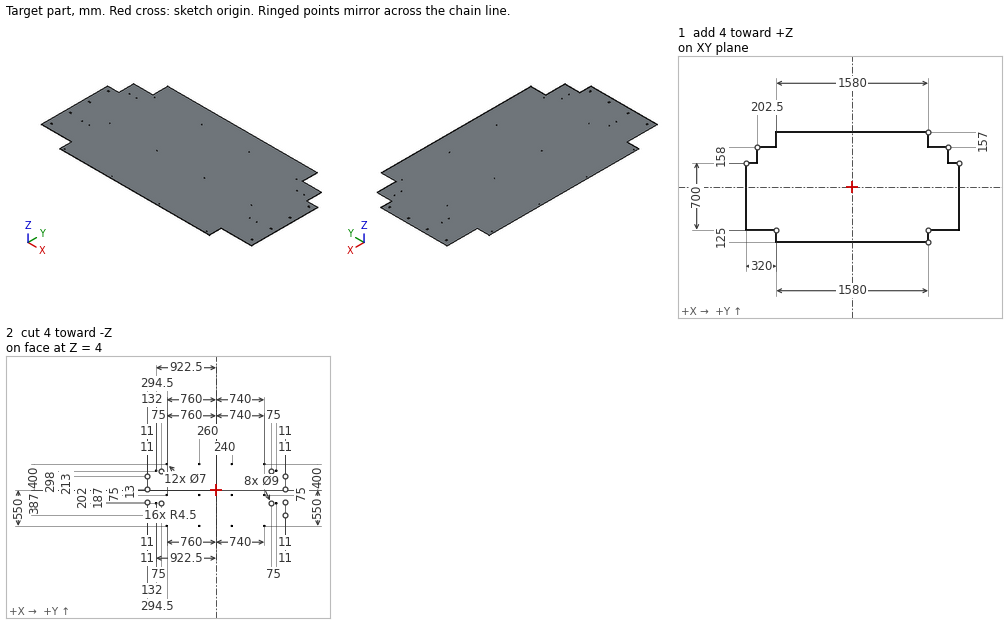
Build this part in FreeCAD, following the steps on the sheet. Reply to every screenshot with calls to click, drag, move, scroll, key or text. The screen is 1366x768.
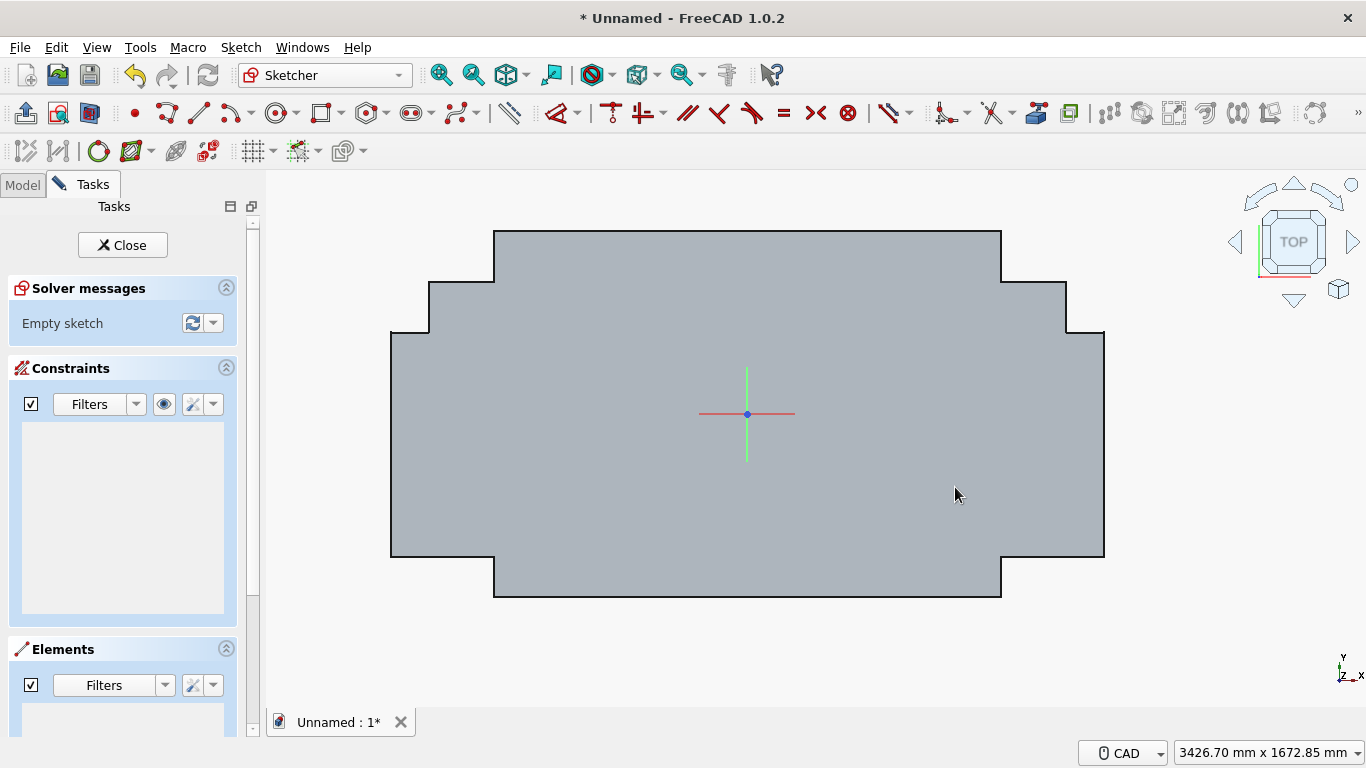
click(412, 114)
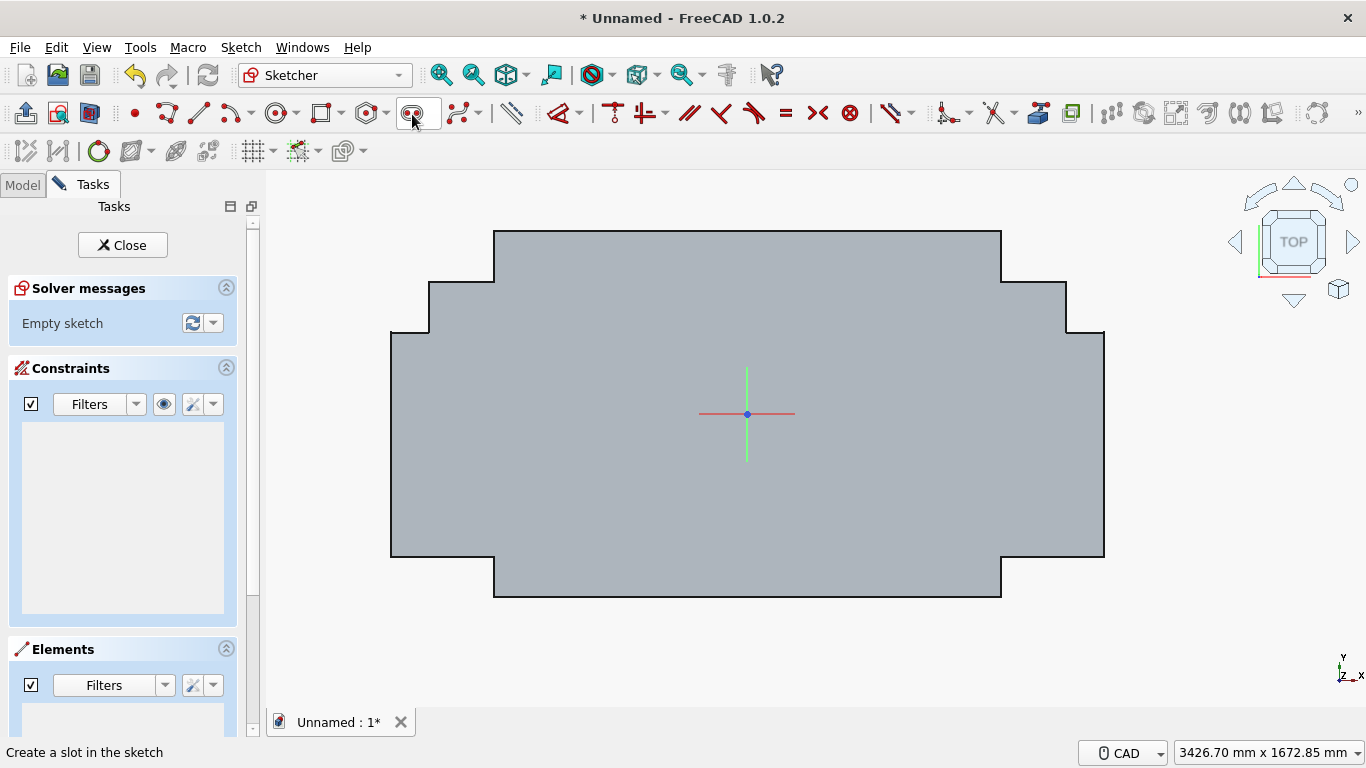
scroll(405, 346, up, 14)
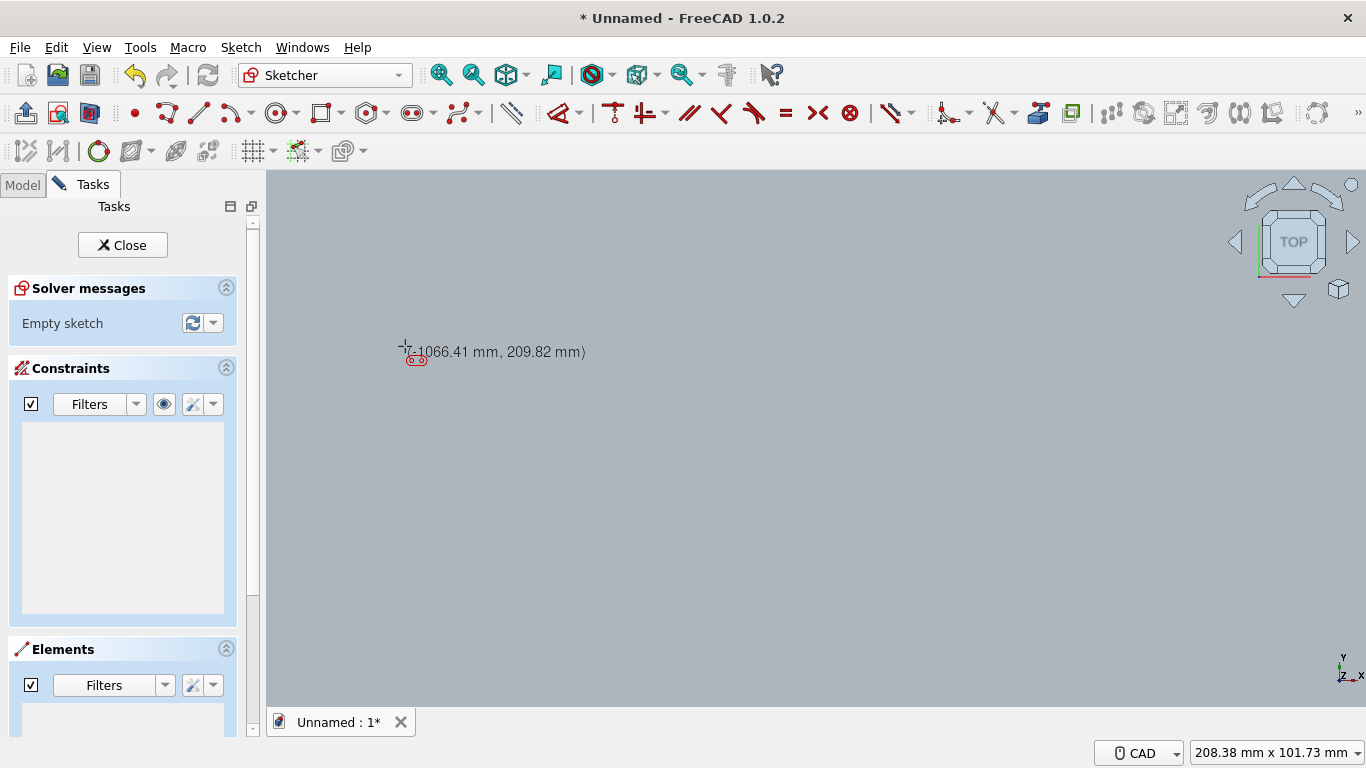
scroll(405, 346, down, 14)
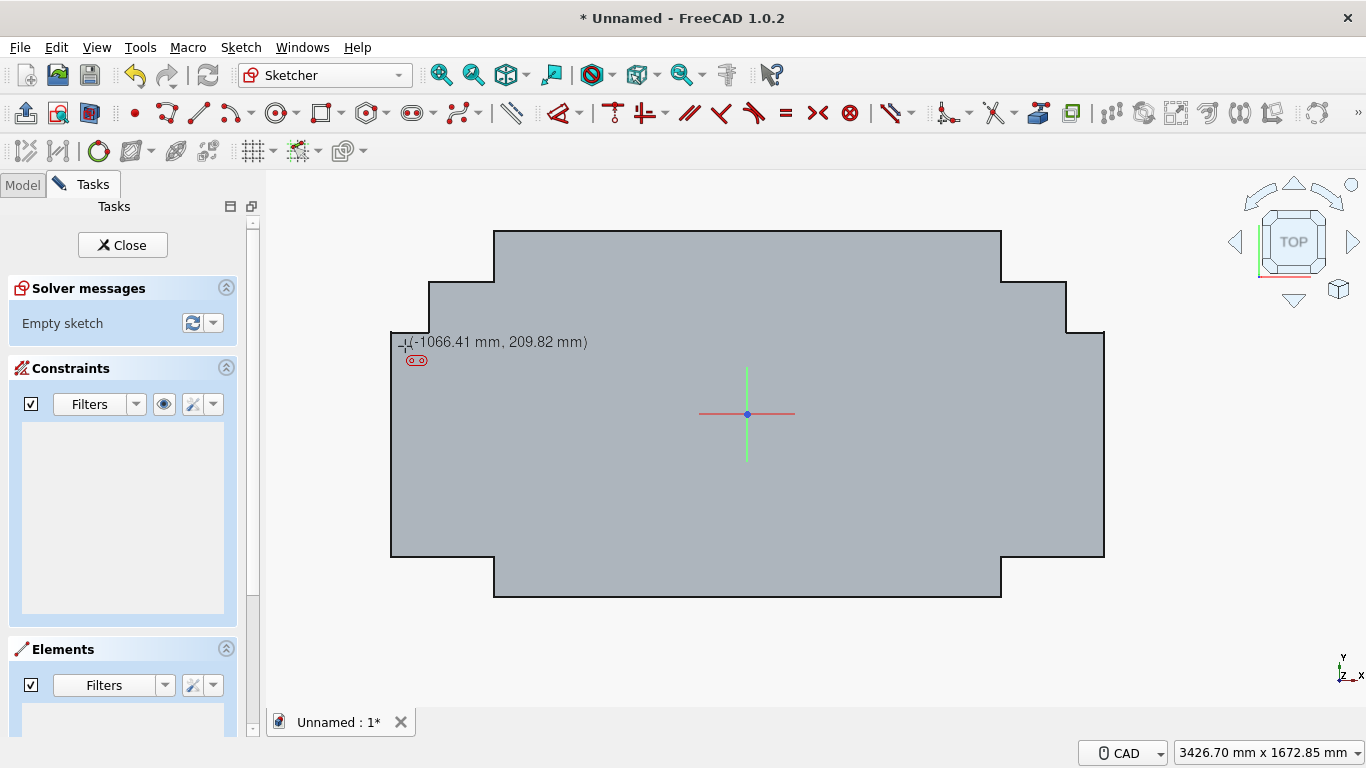
click(405, 346)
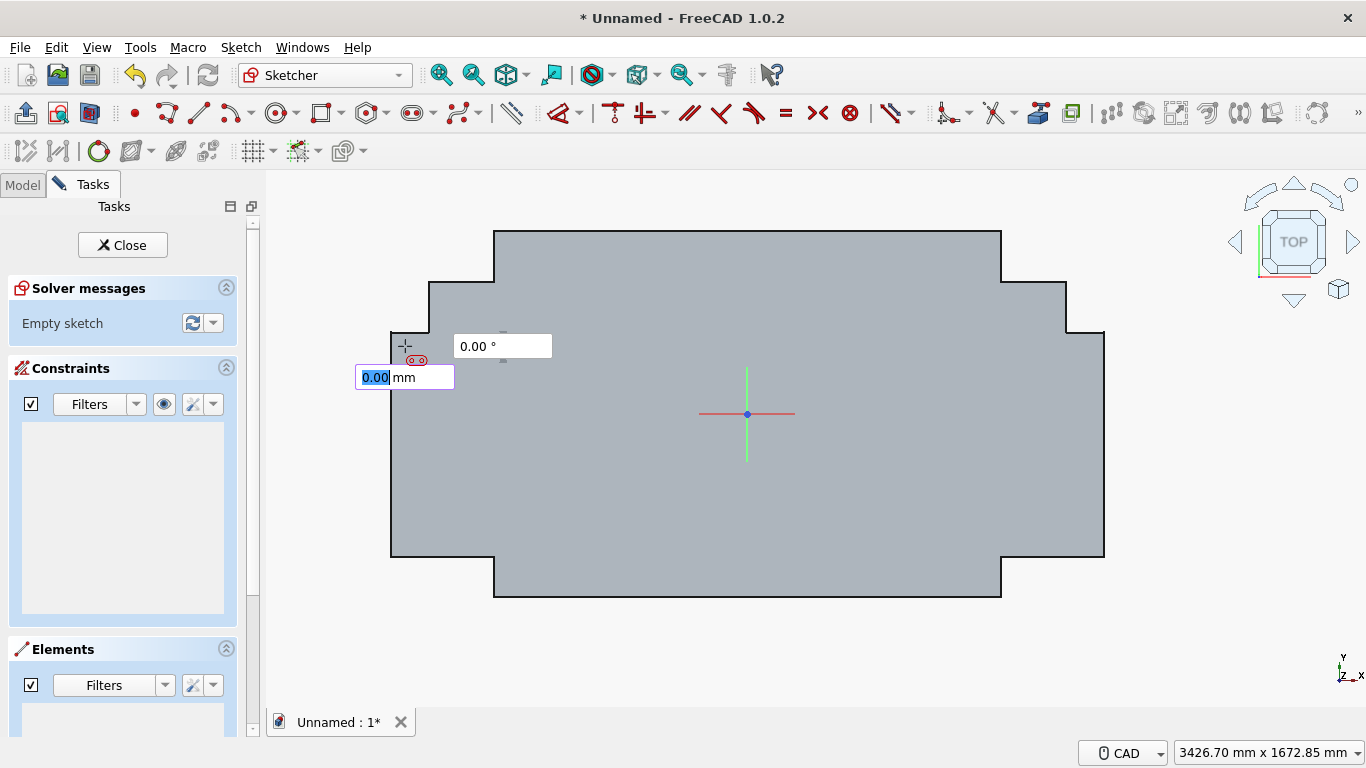
scroll(409, 346, up, 8)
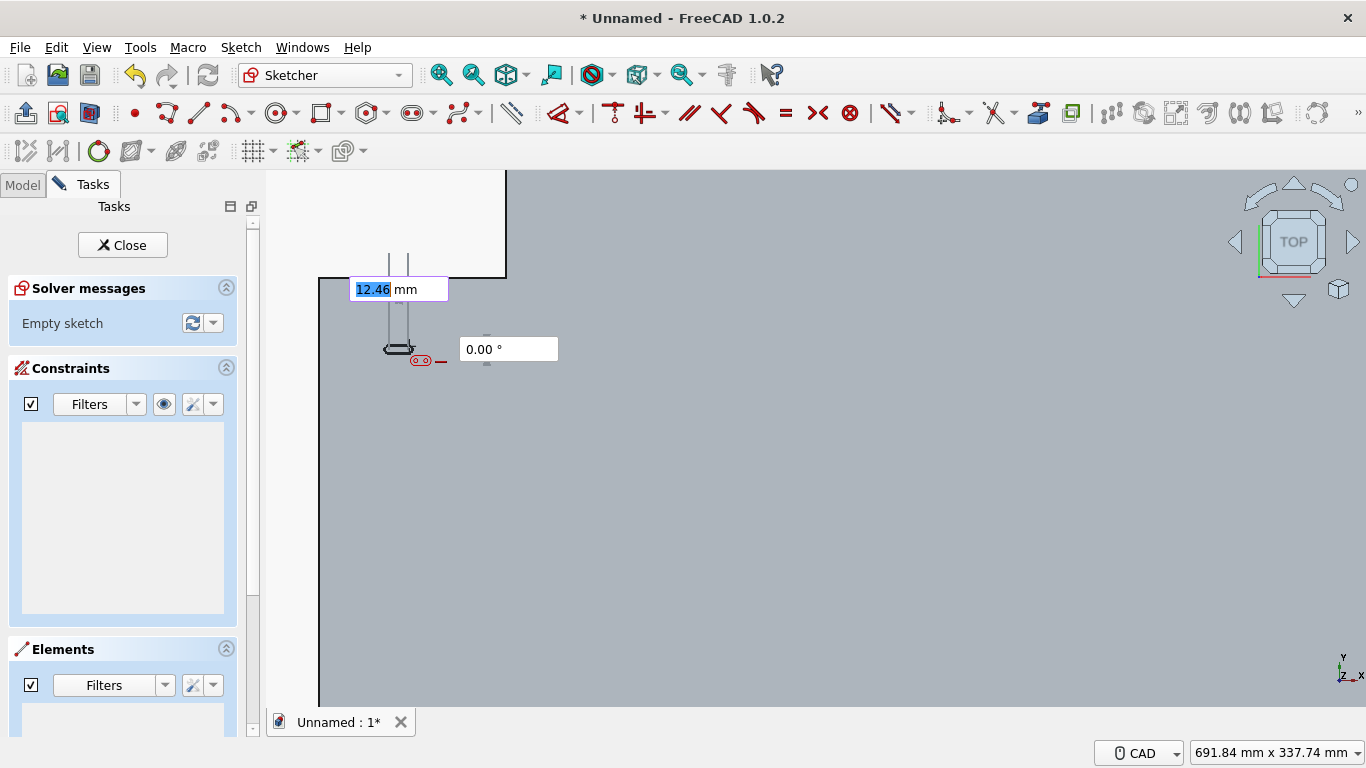
click(408, 345)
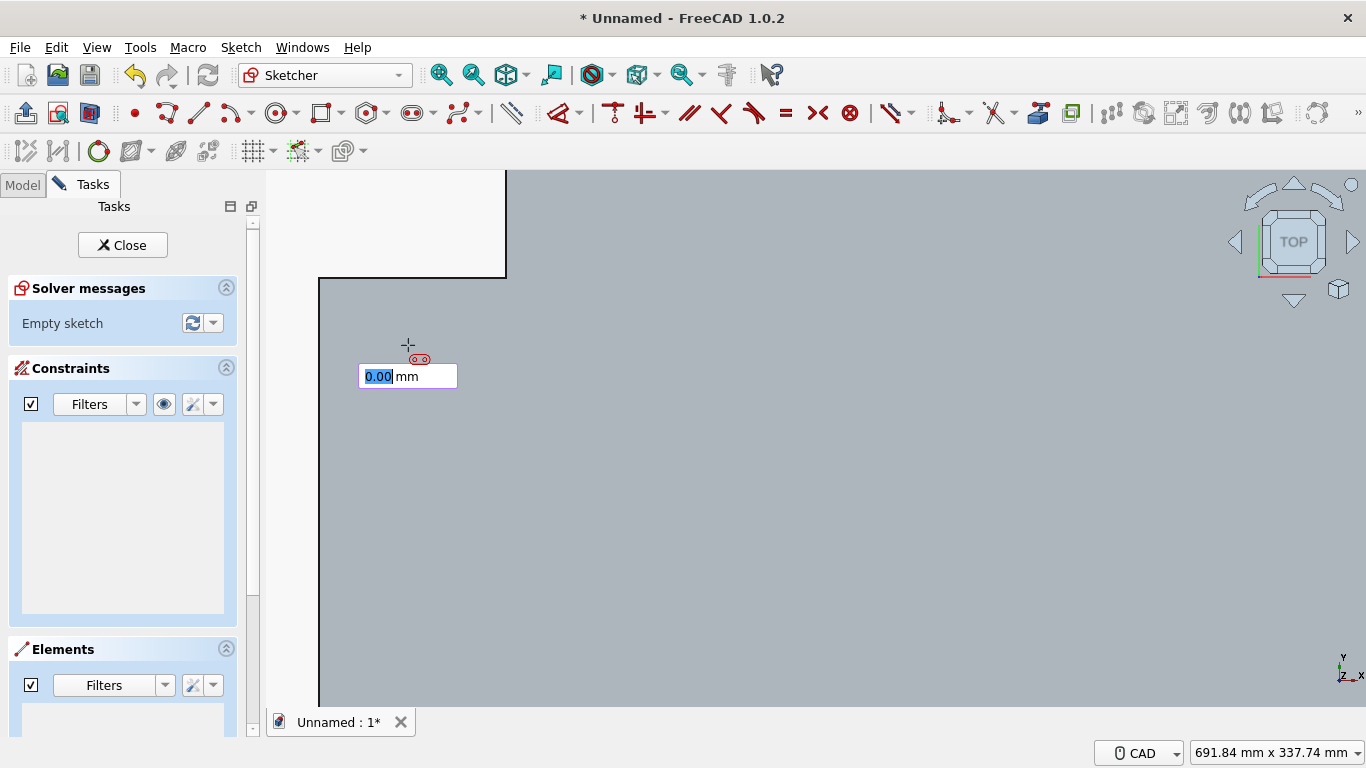
scroll(399, 337, up, 4)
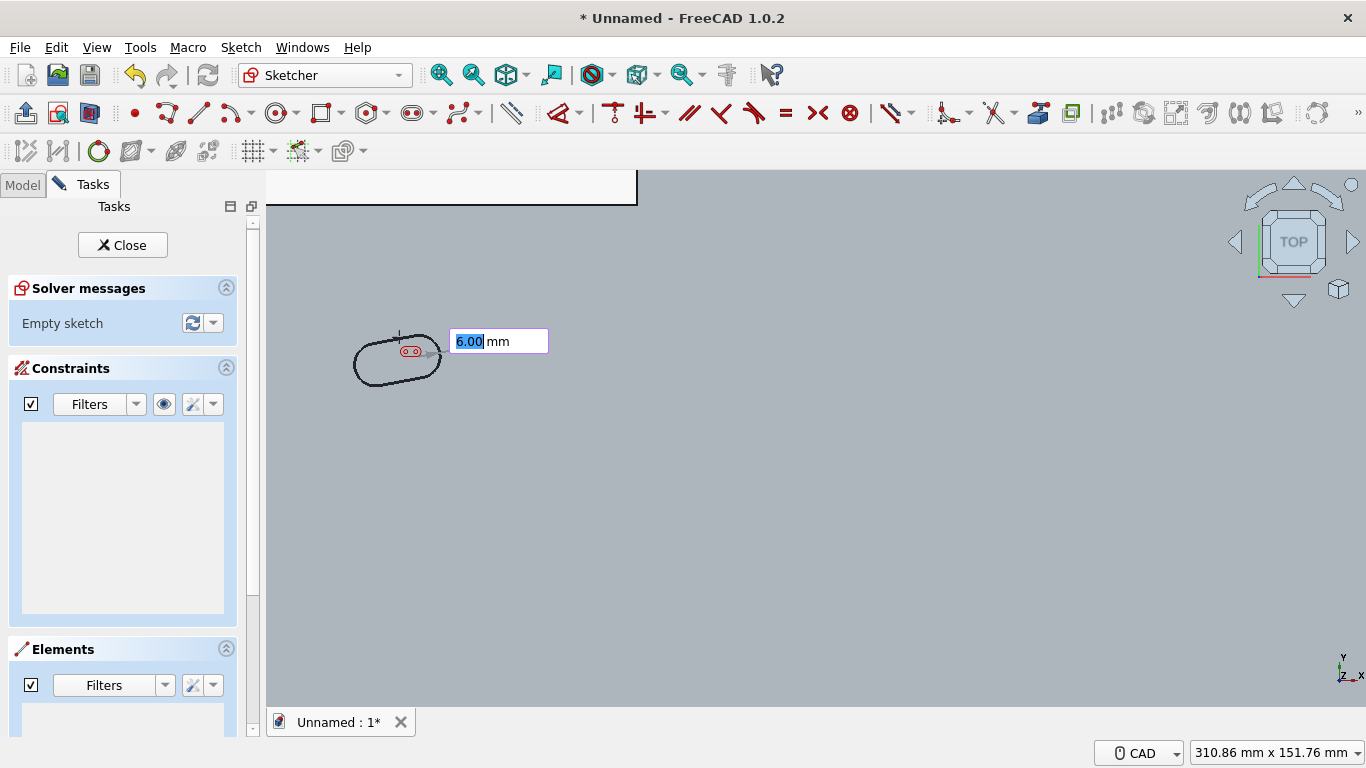
click(399, 338)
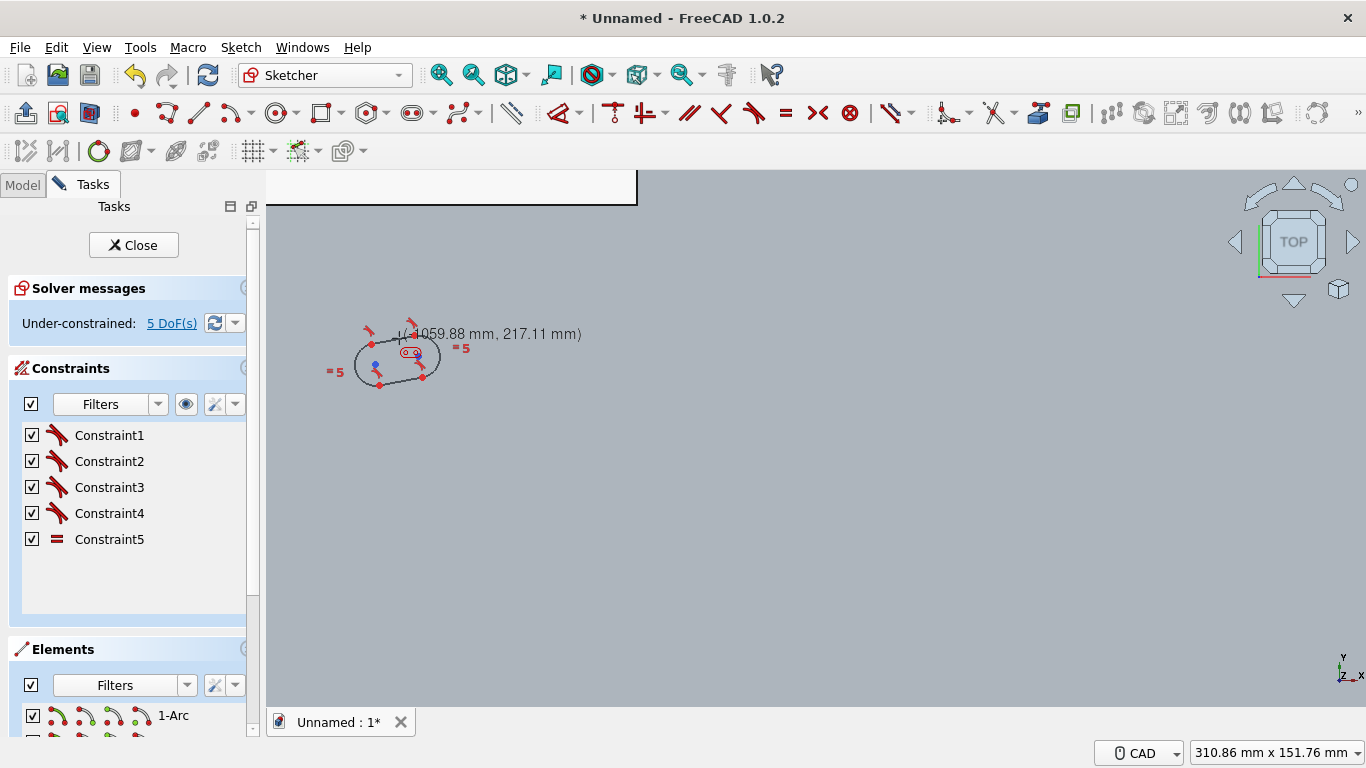
scroll(408, 345, down, 12)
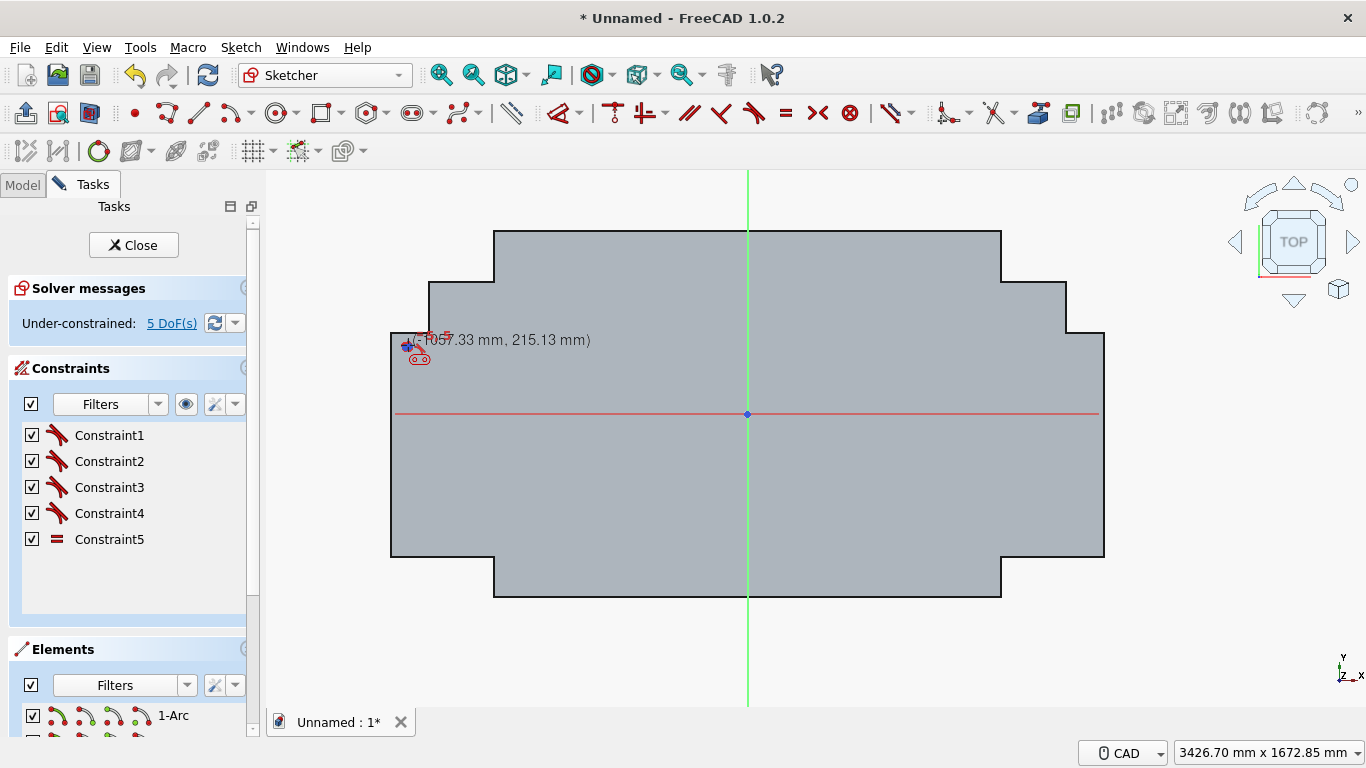
scroll(405, 410, up, 14)